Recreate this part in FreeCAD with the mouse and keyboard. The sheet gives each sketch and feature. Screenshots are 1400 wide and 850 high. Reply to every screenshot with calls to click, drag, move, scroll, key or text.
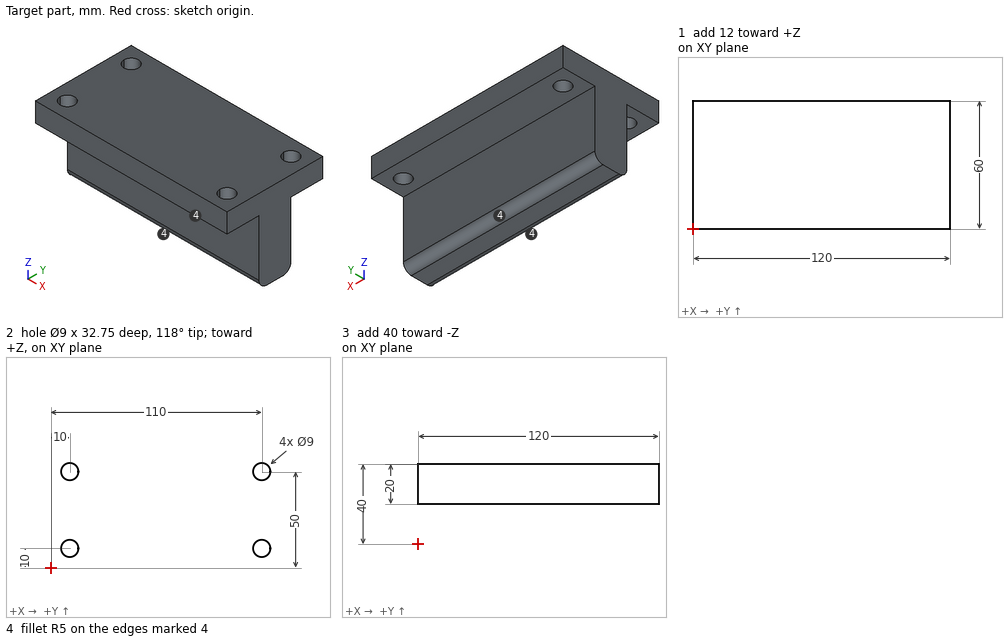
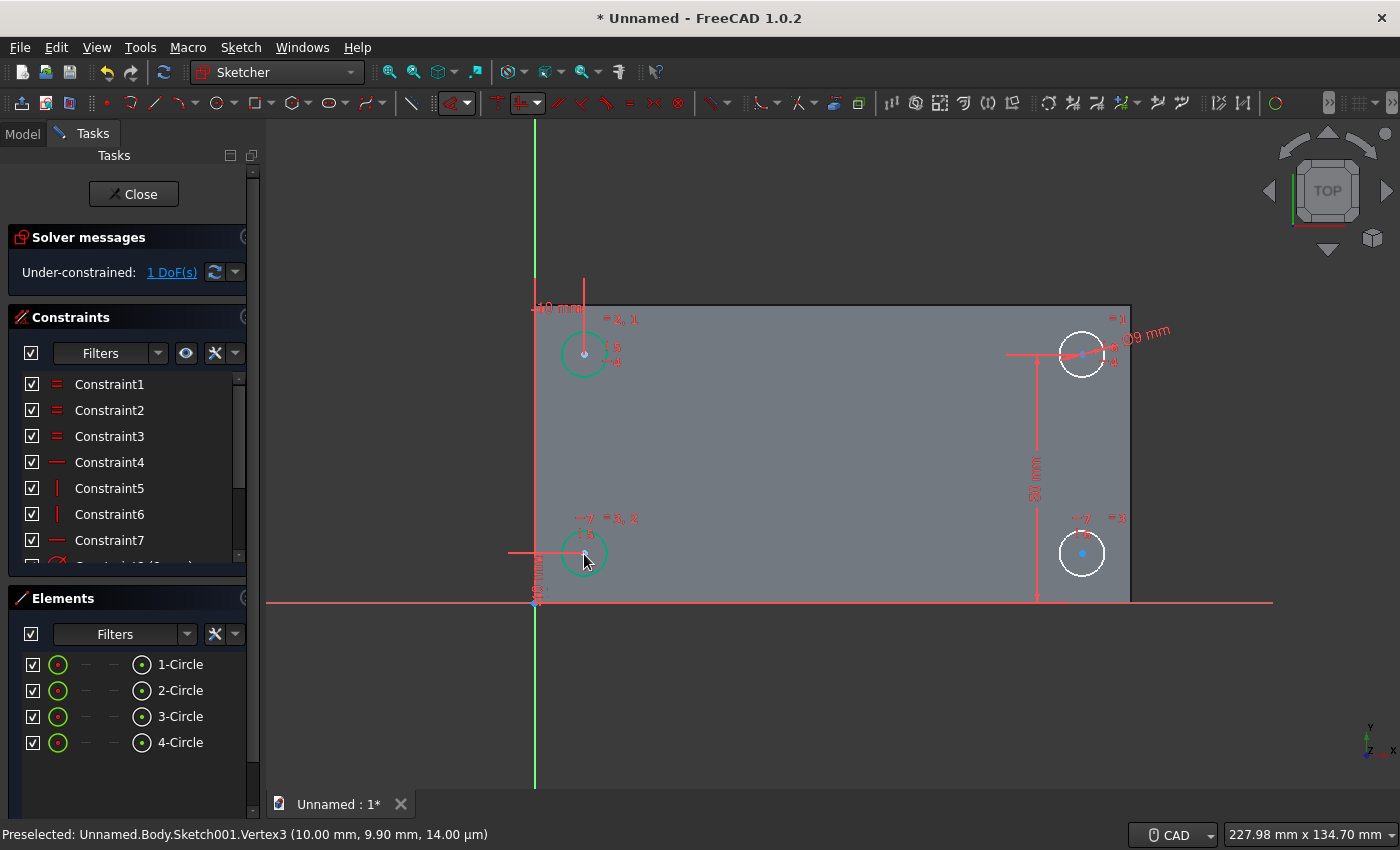
click(1082, 355)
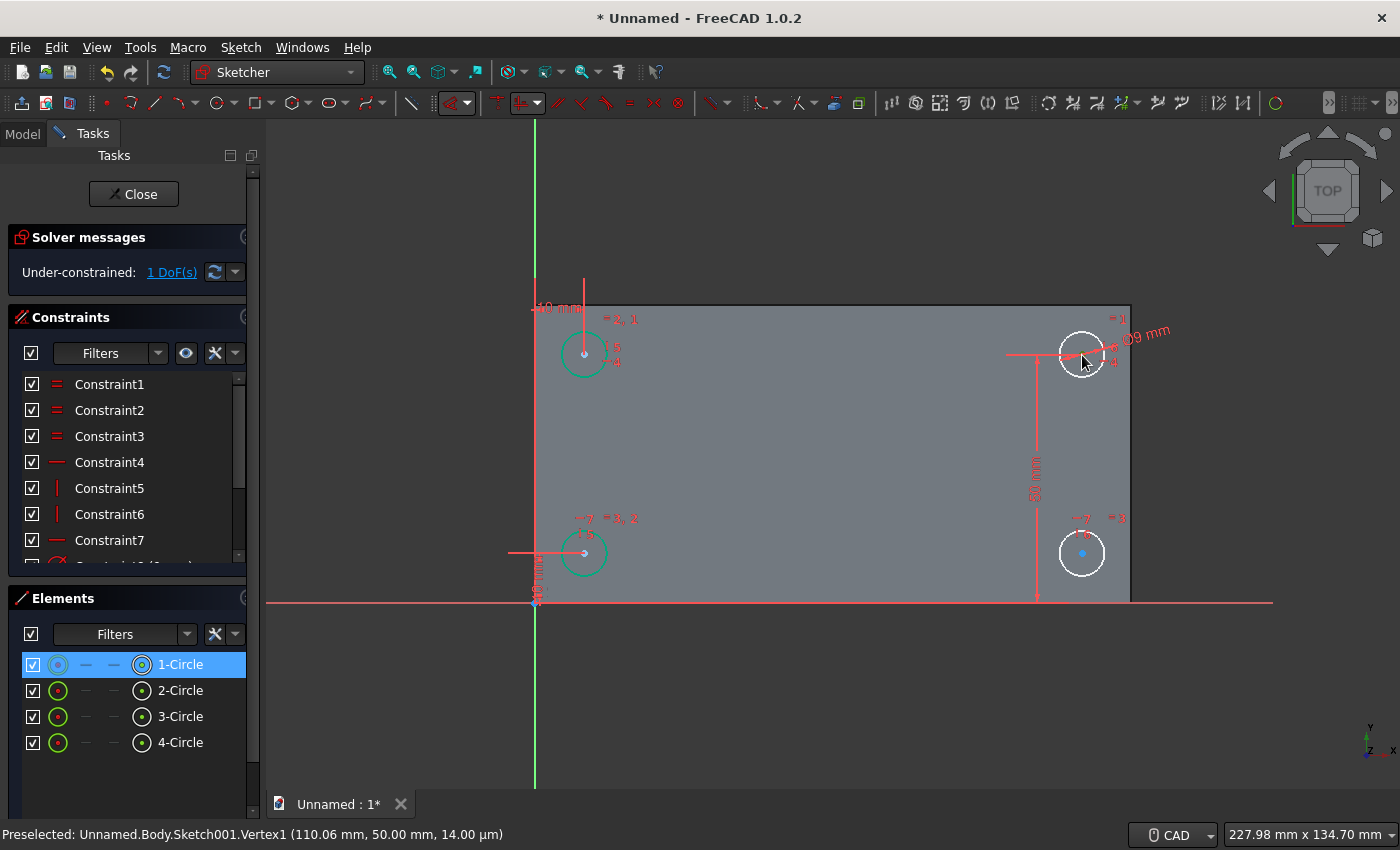
click(470, 104)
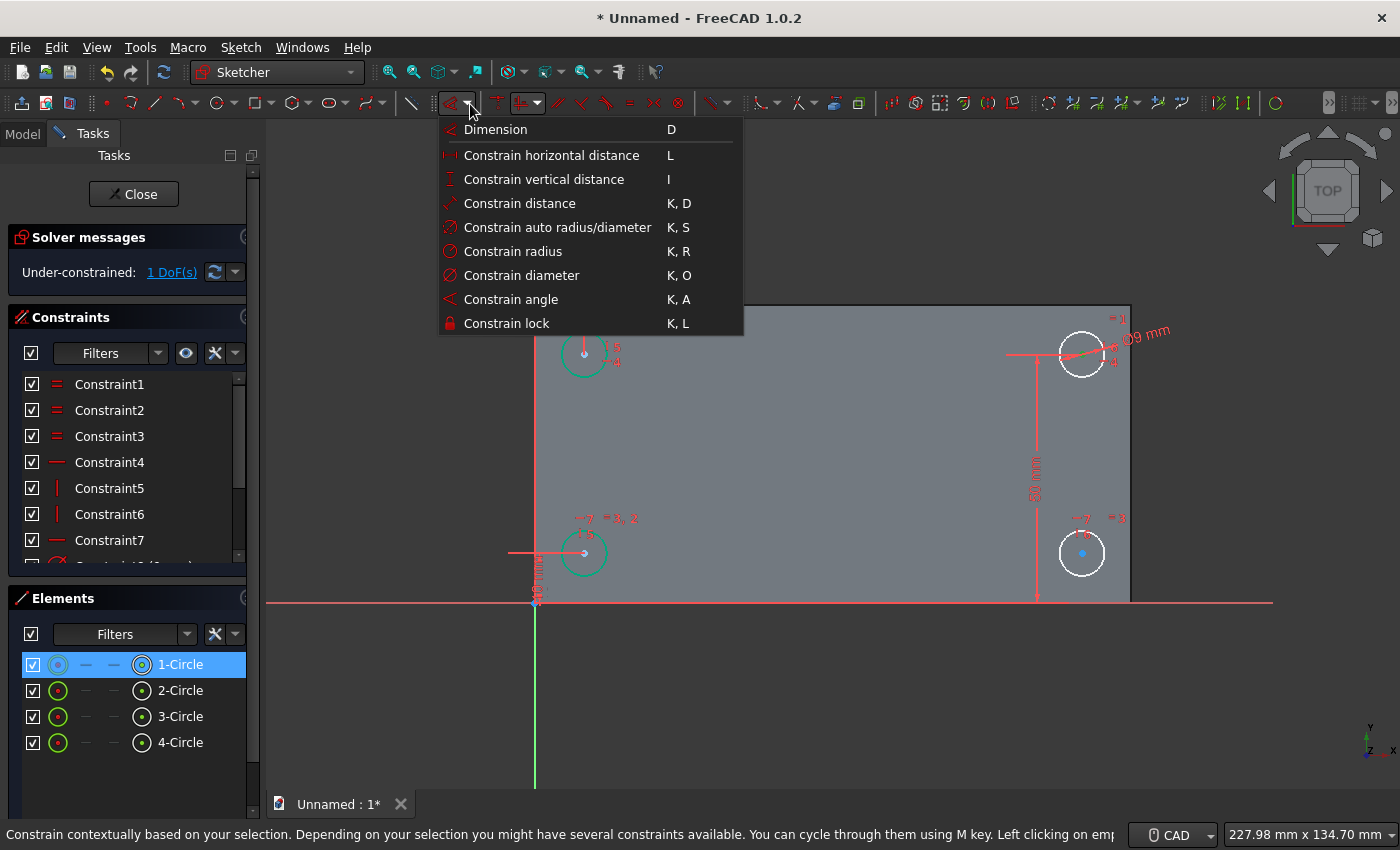
click(591, 155)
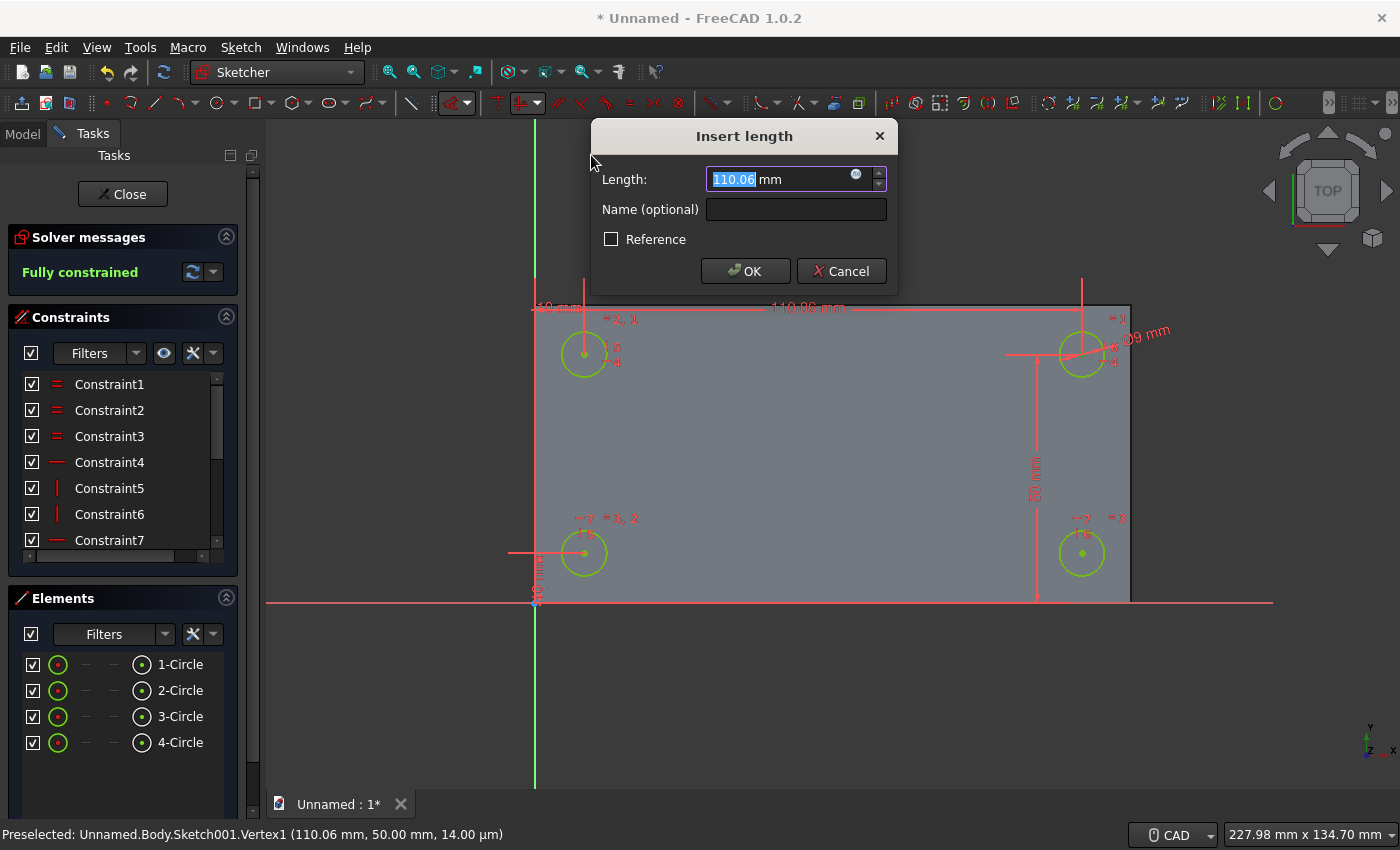
text(110)
key(Return)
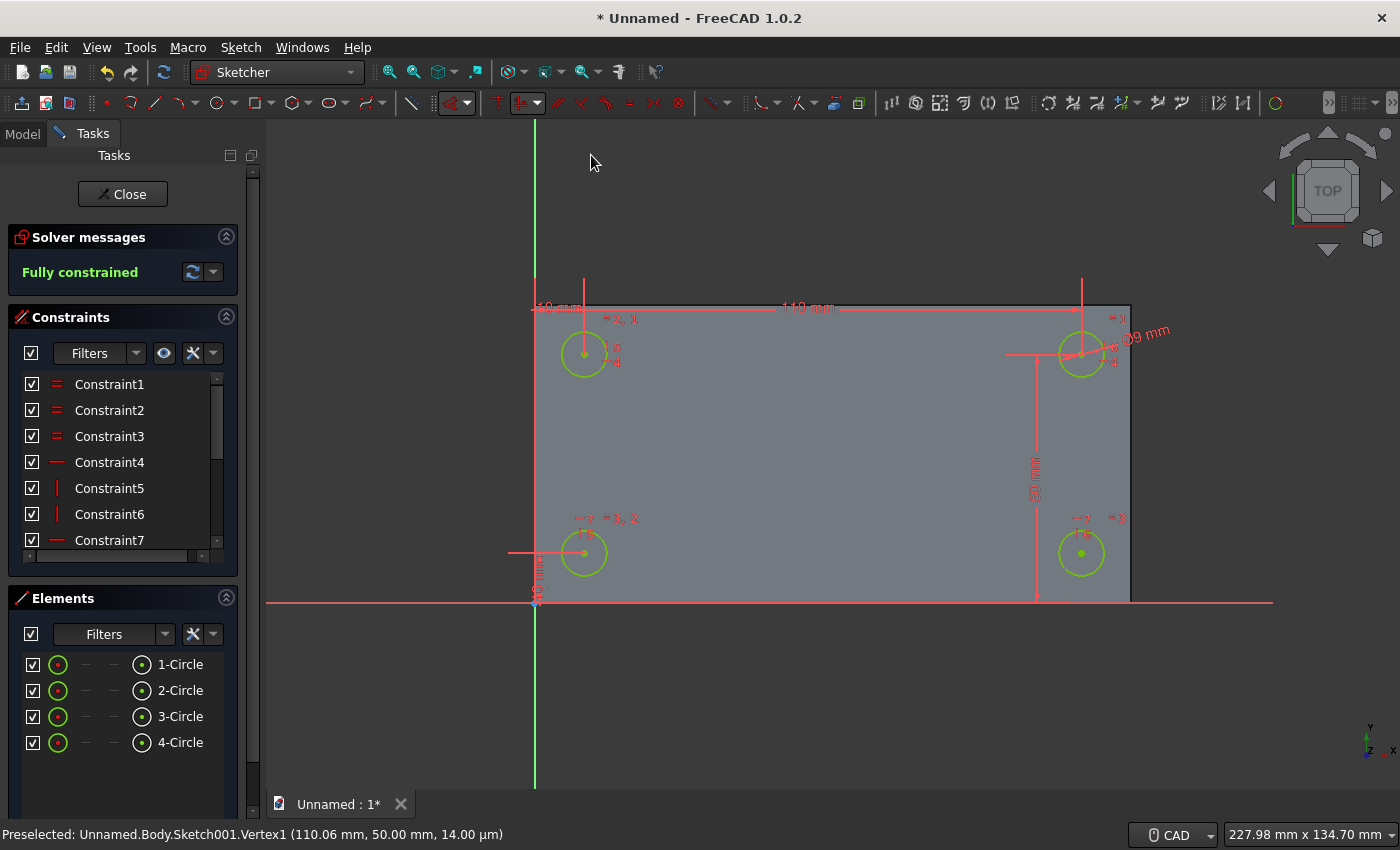
click(123, 194)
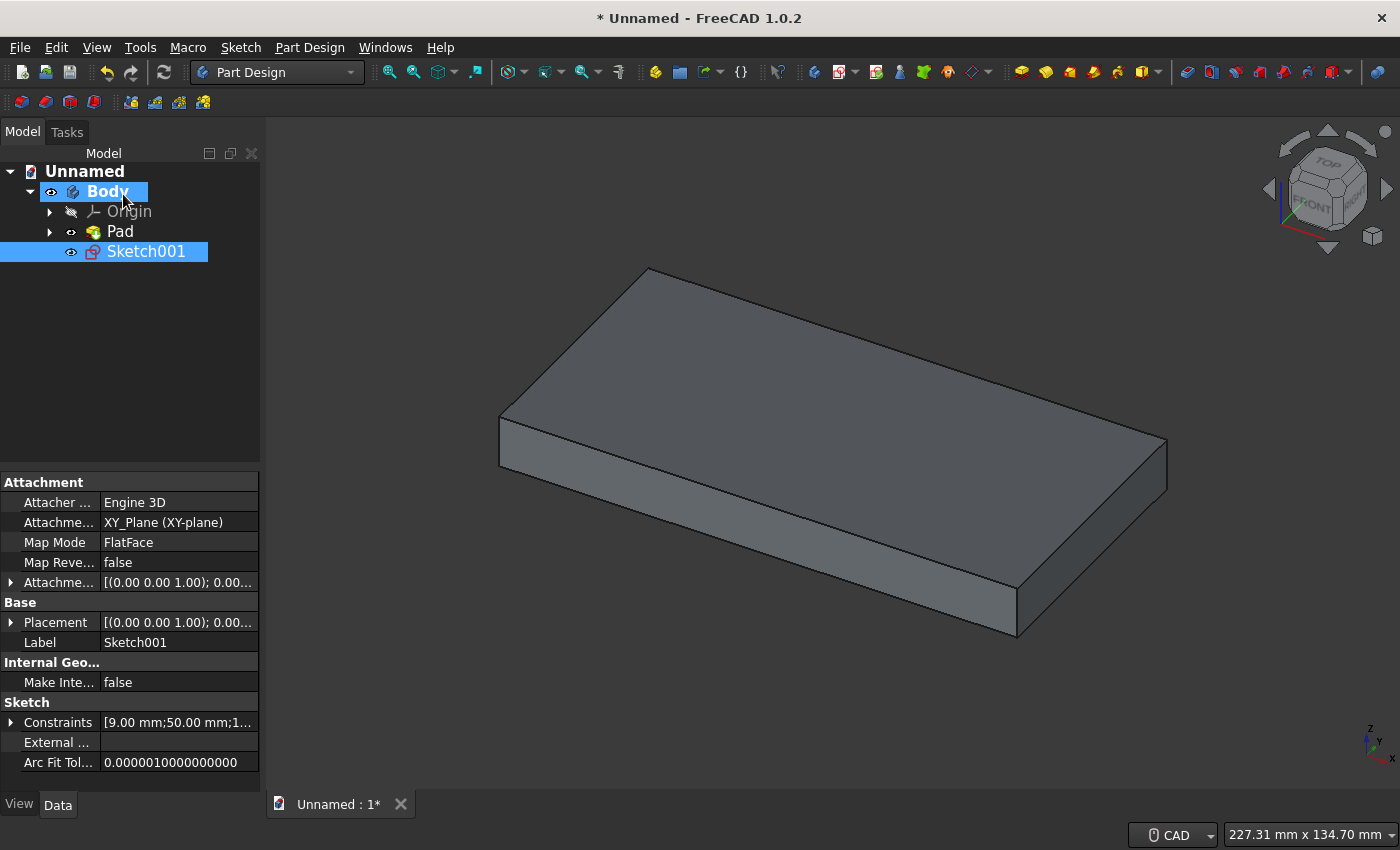
click(1212, 72)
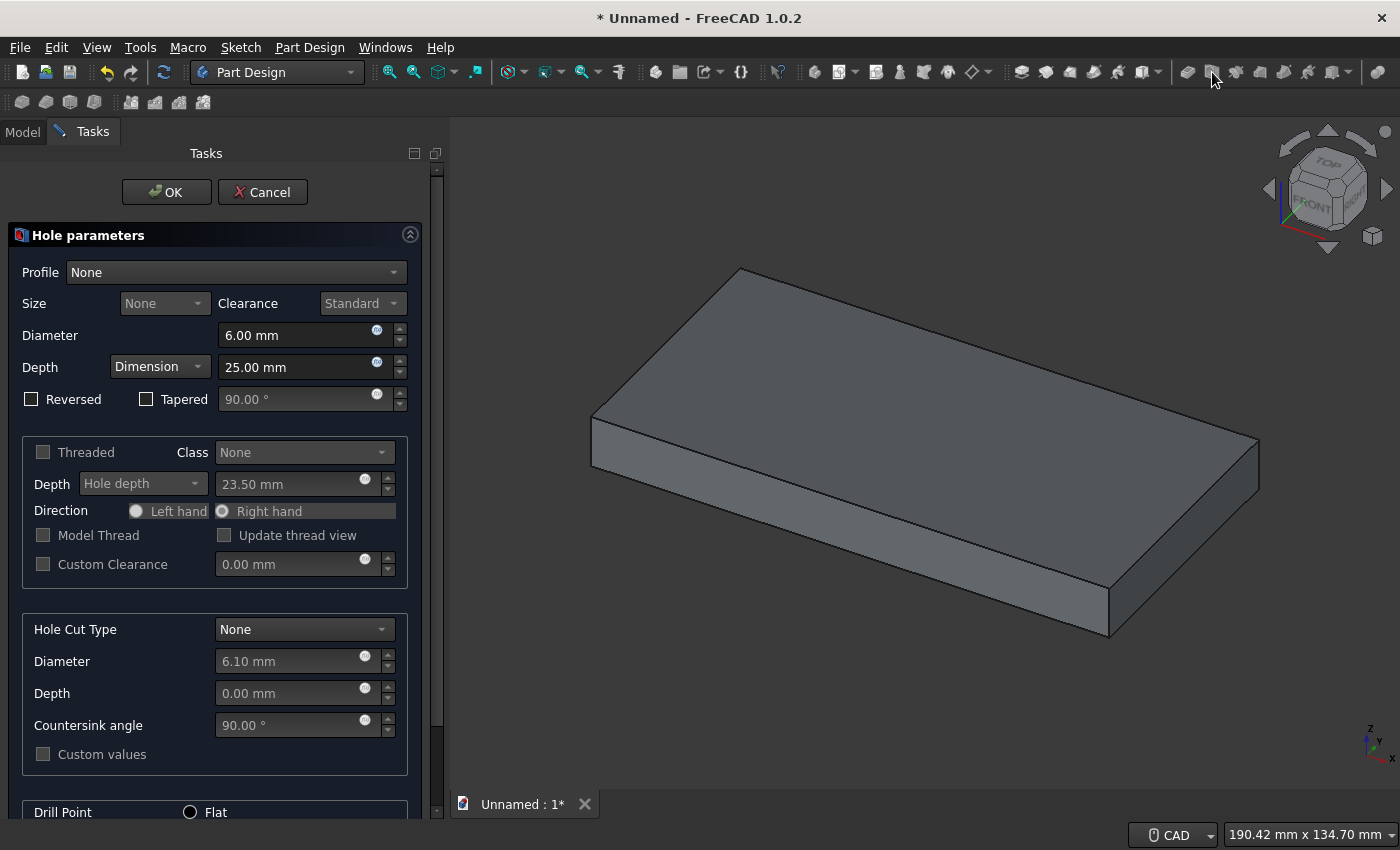
triple_click(305, 335)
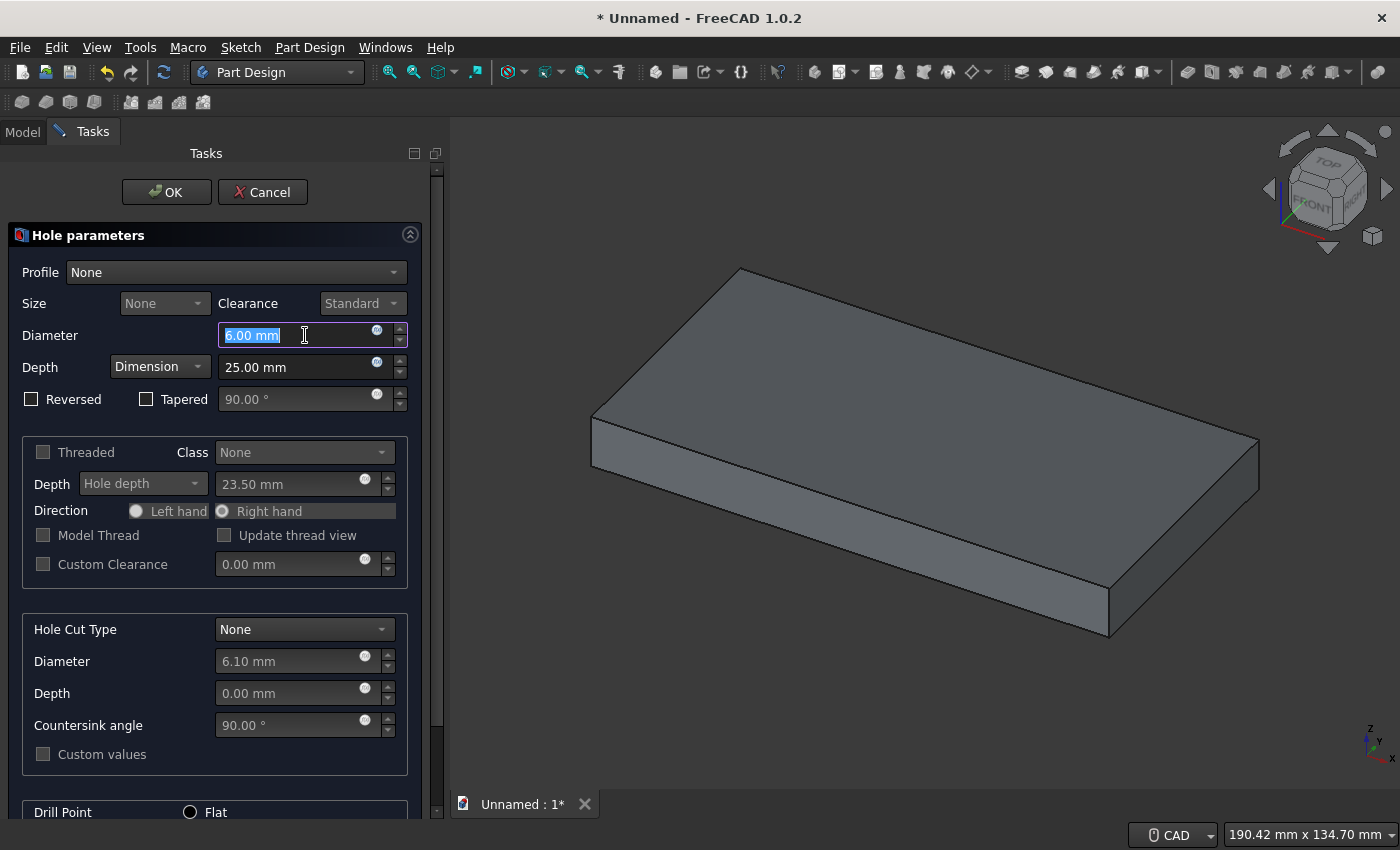
text(9)
key(Tab)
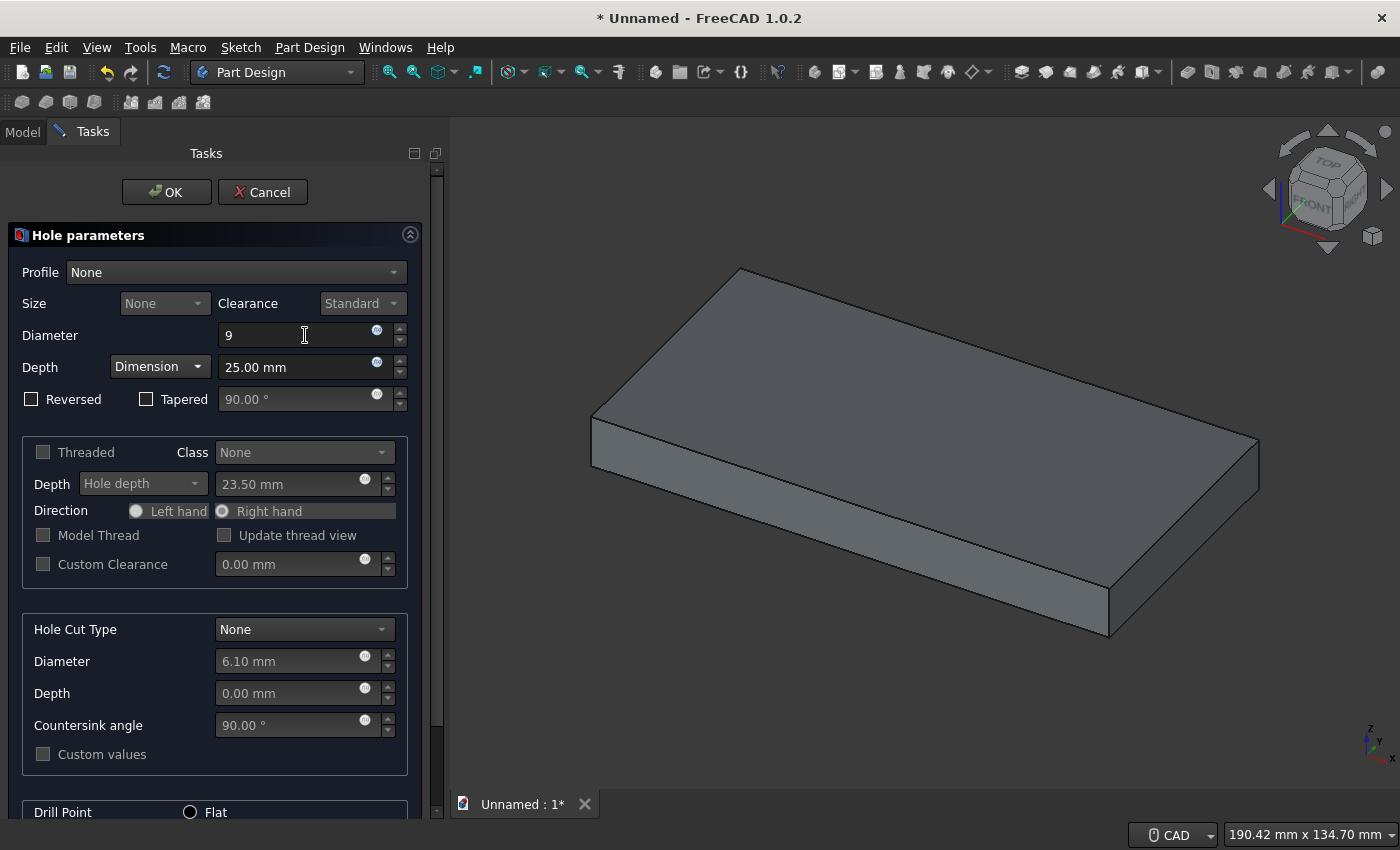
triple_click(305, 367)